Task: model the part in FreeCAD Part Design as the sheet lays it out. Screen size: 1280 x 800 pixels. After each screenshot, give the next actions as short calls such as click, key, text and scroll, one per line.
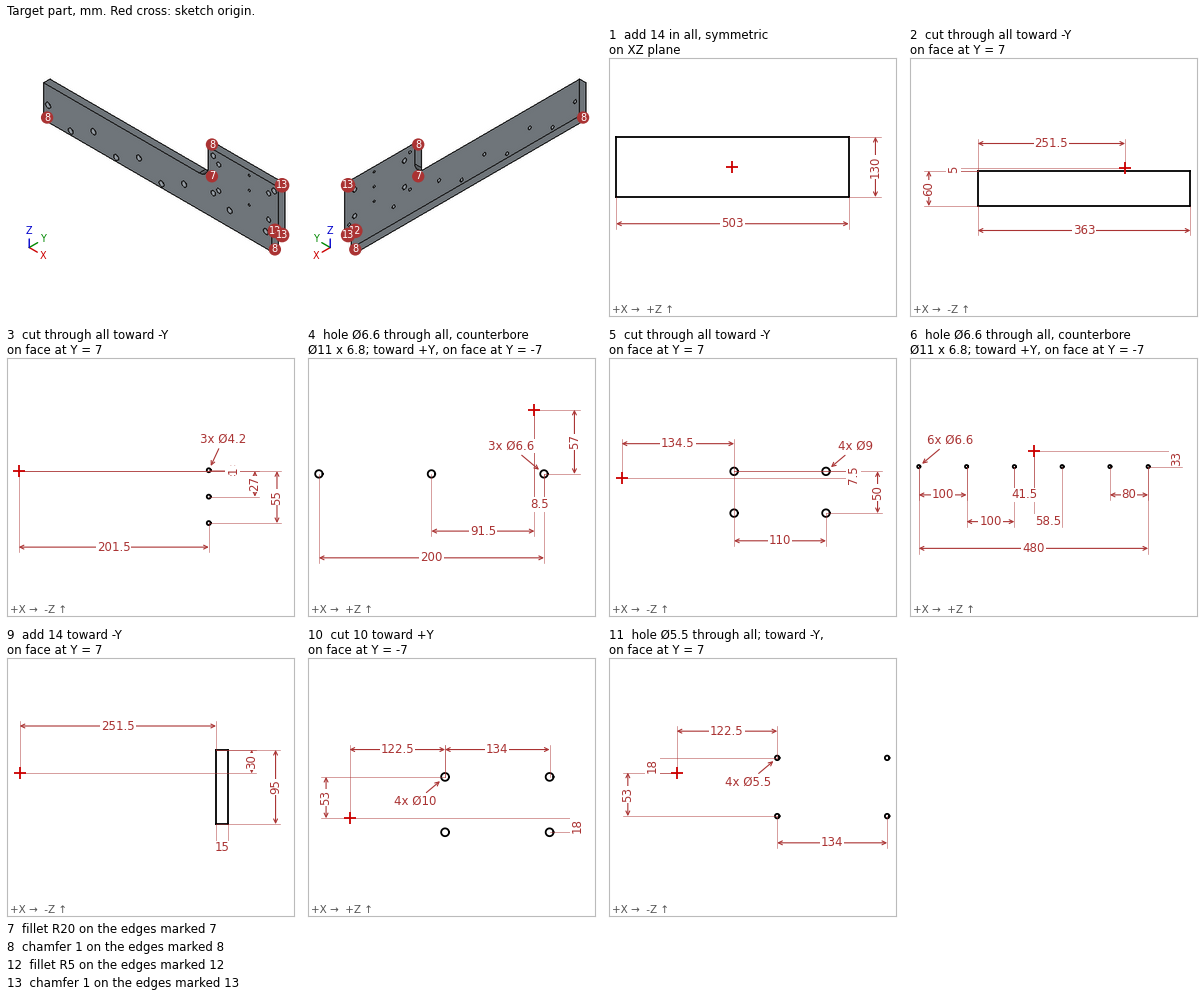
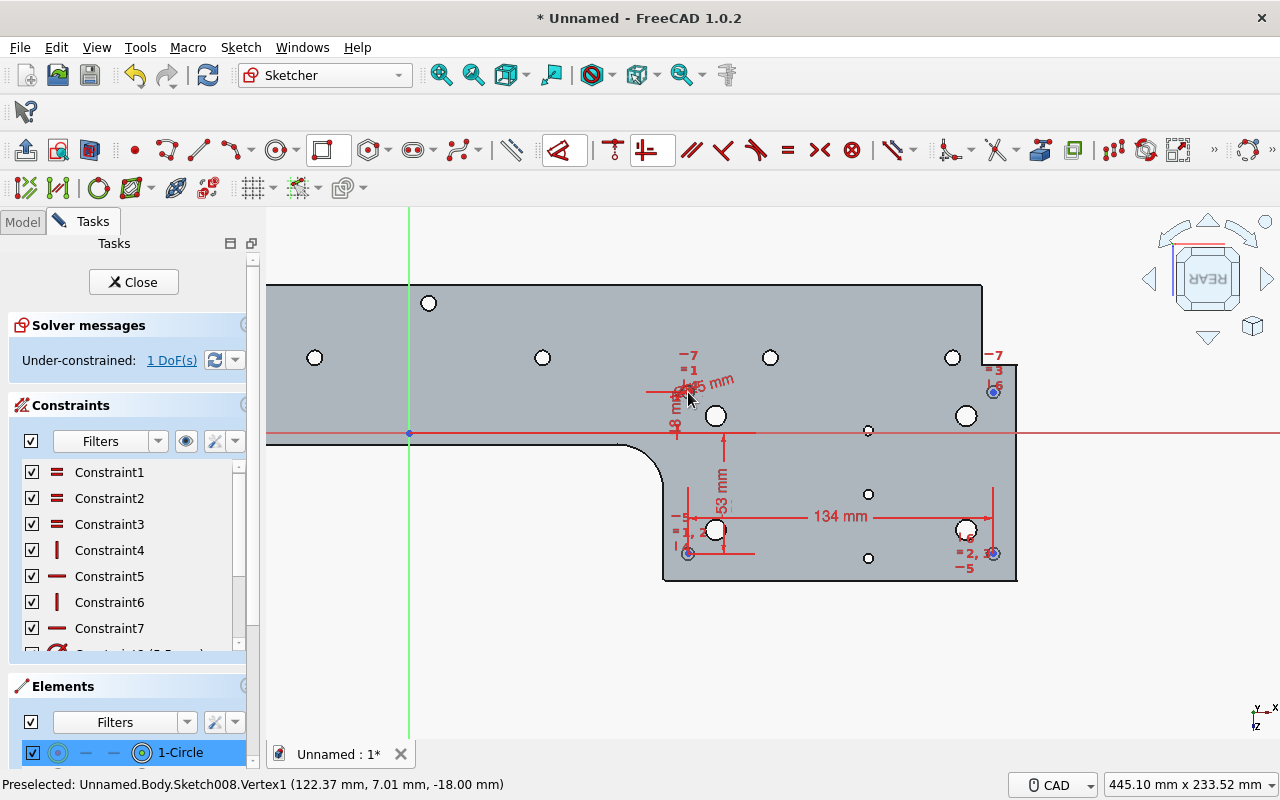
key(l)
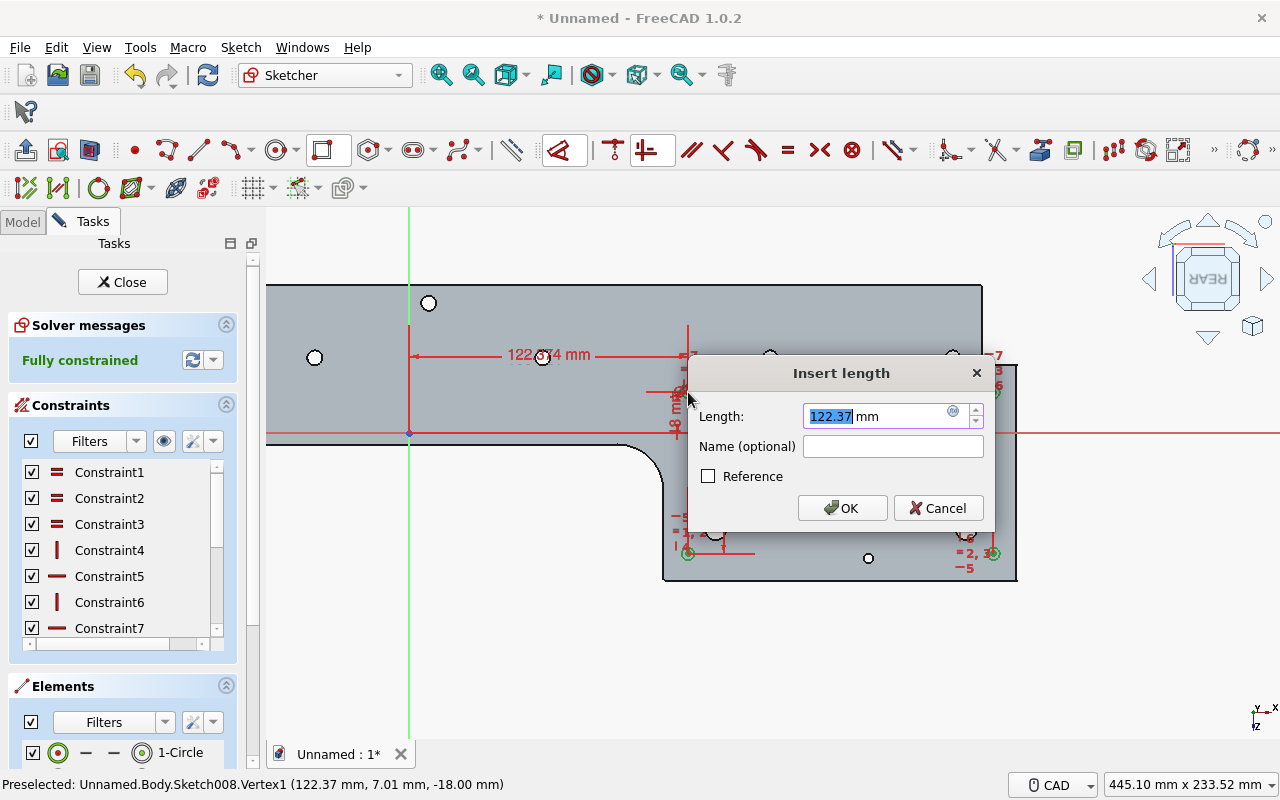
text(122.5)
key(Return)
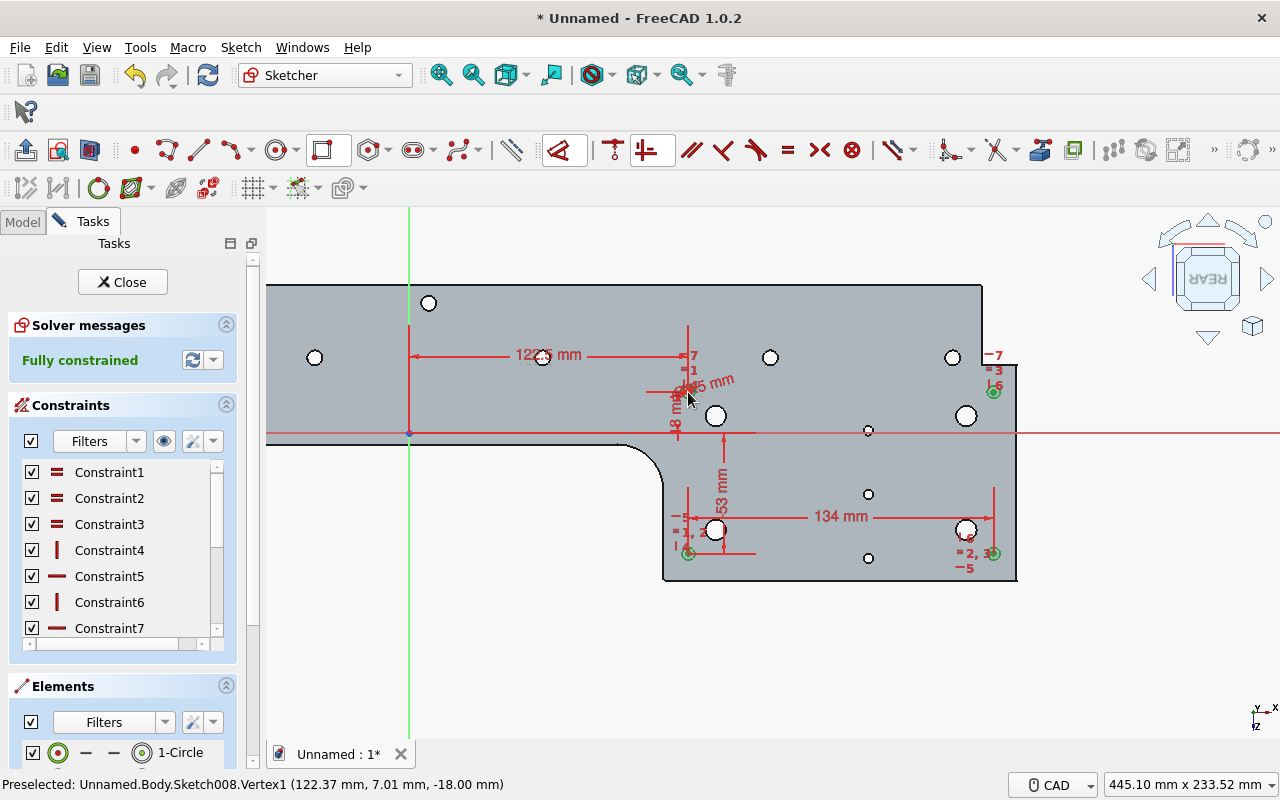
click(123, 282)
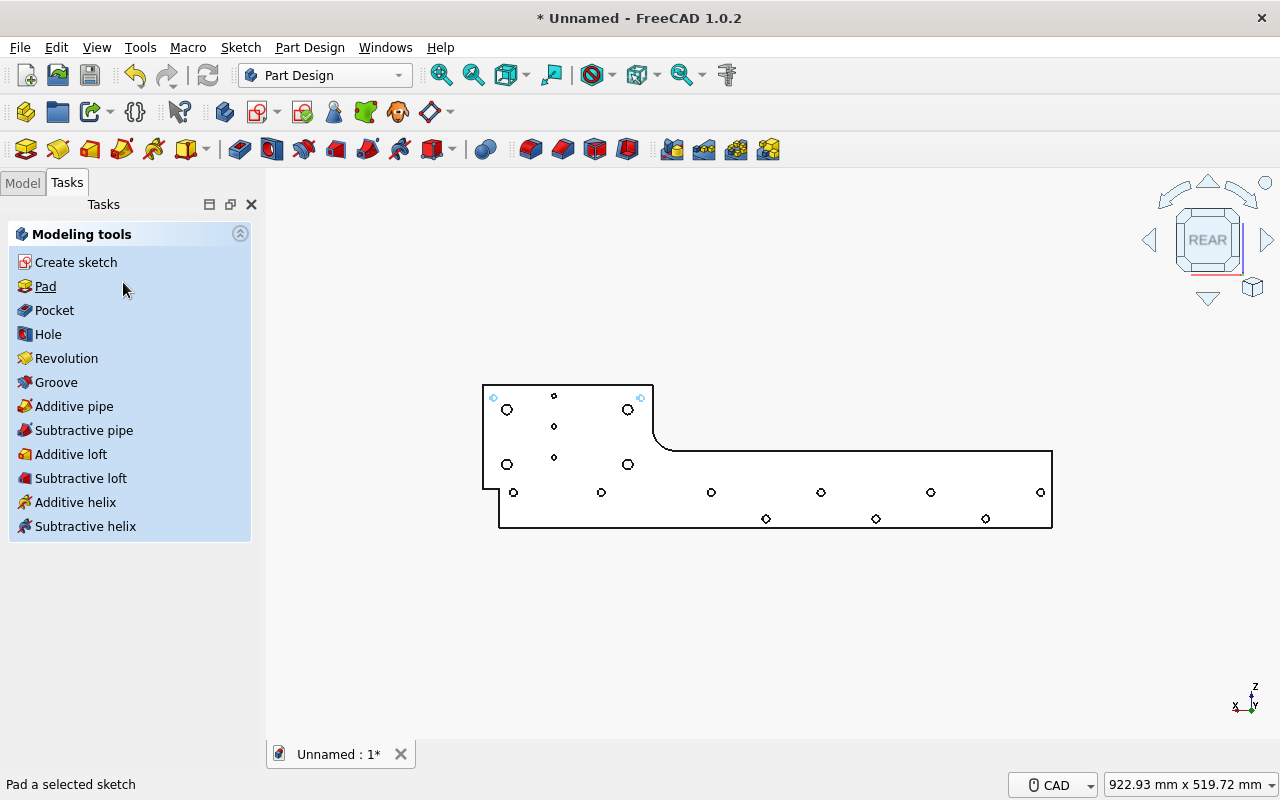
click(272, 150)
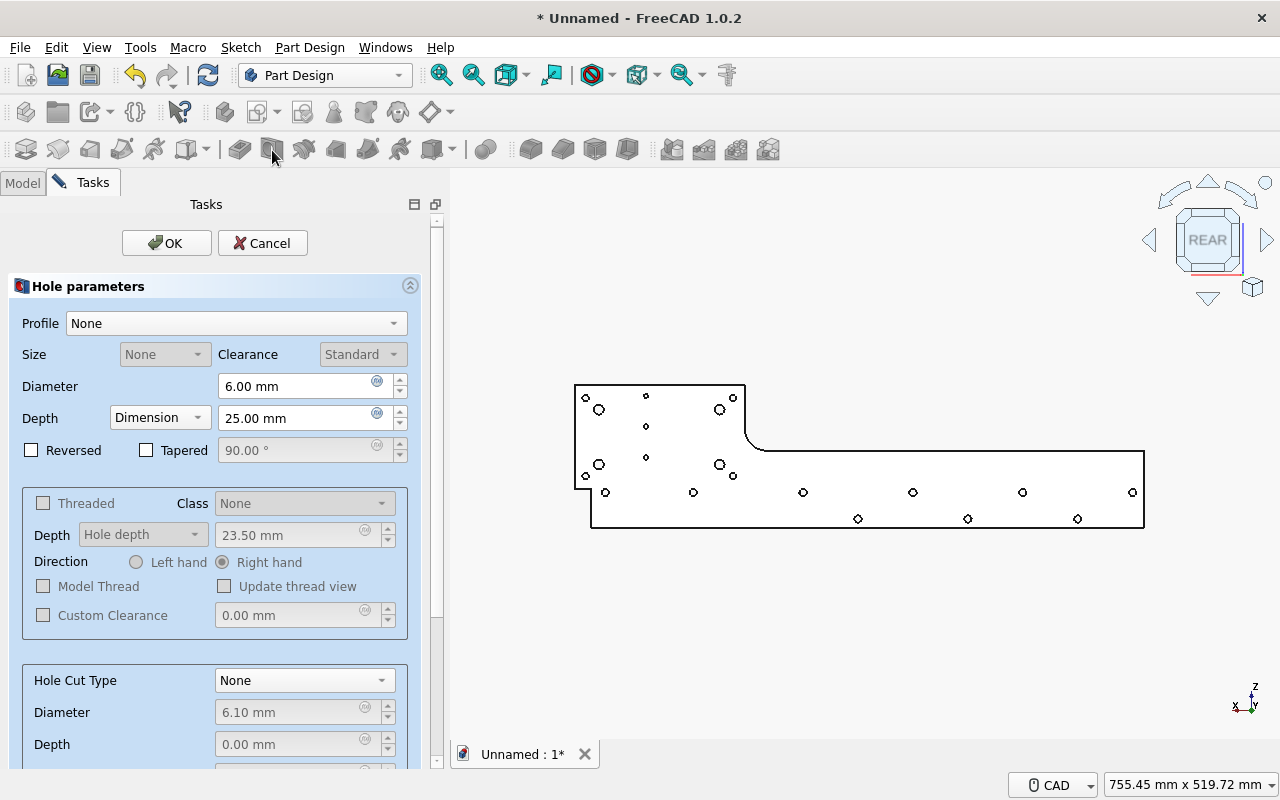
triple_click(305, 386)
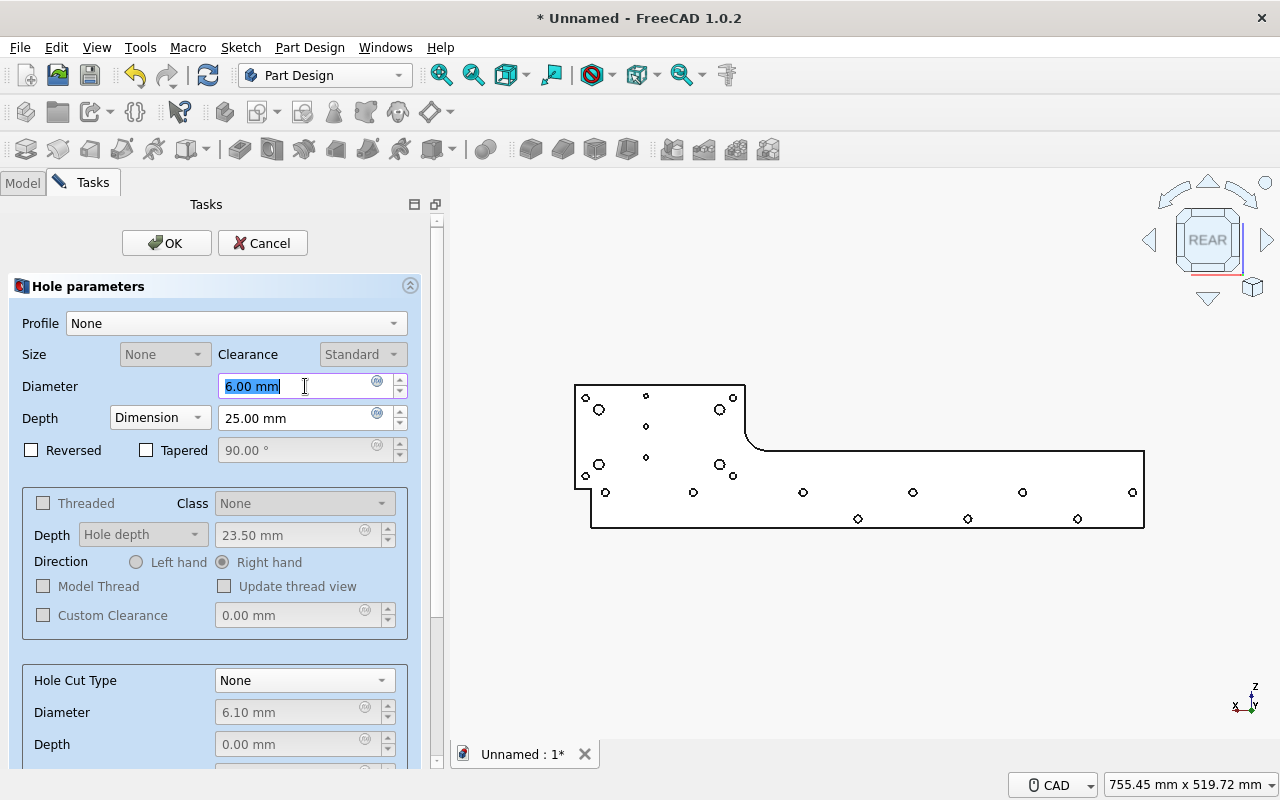
text(5.5)
key(Tab)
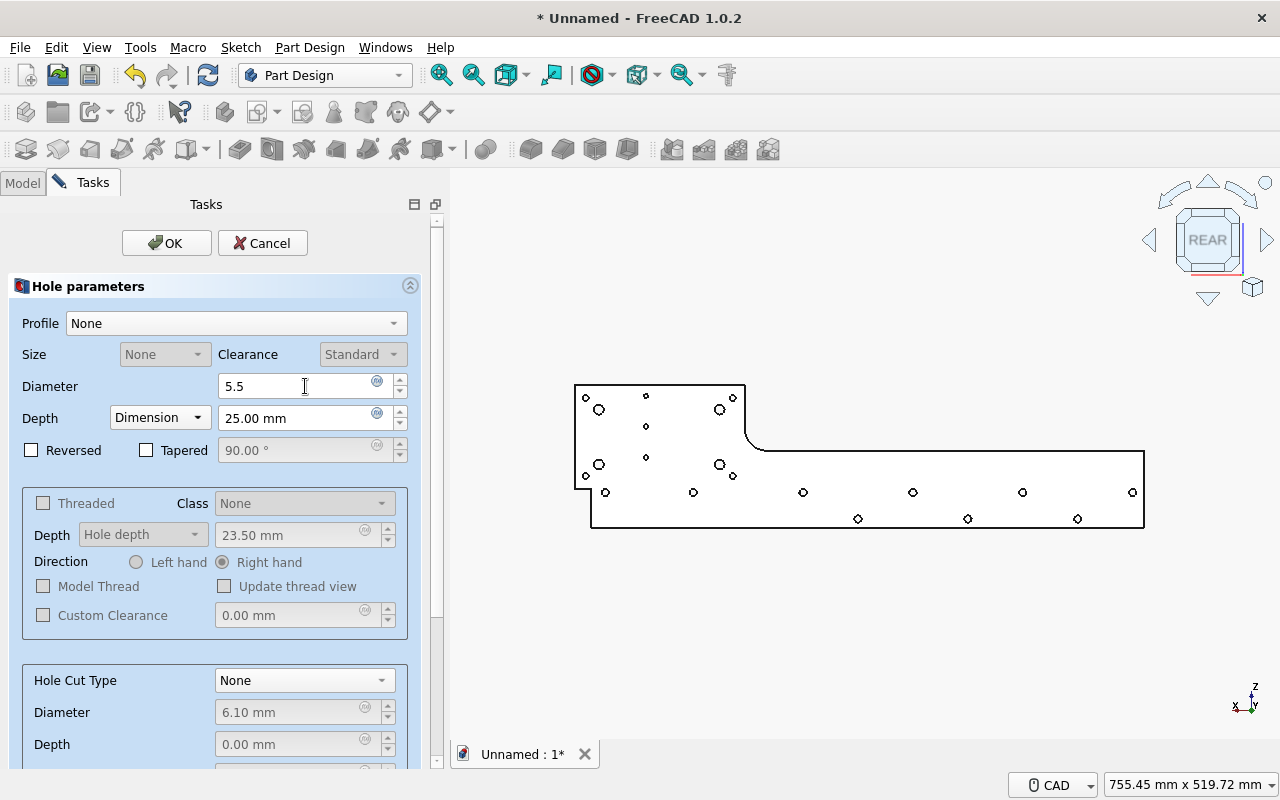
click(161, 418)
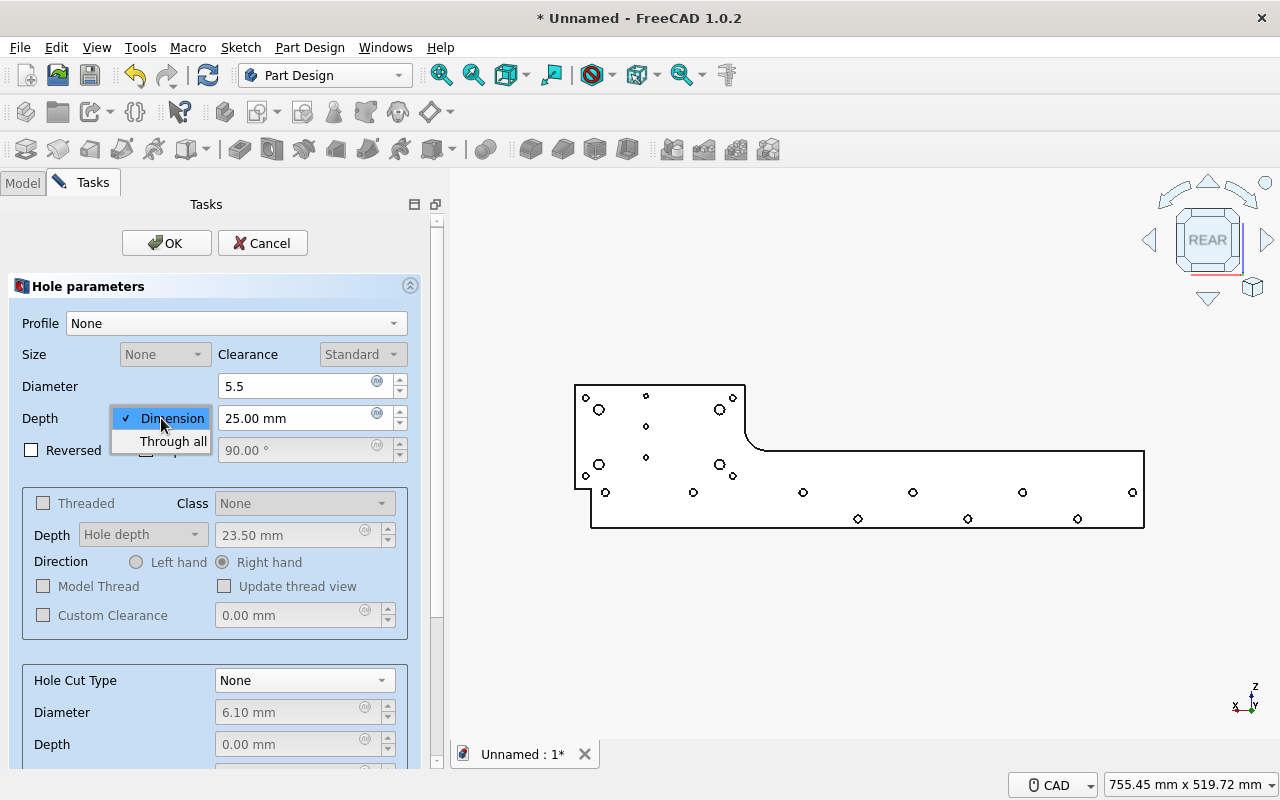
click(160, 442)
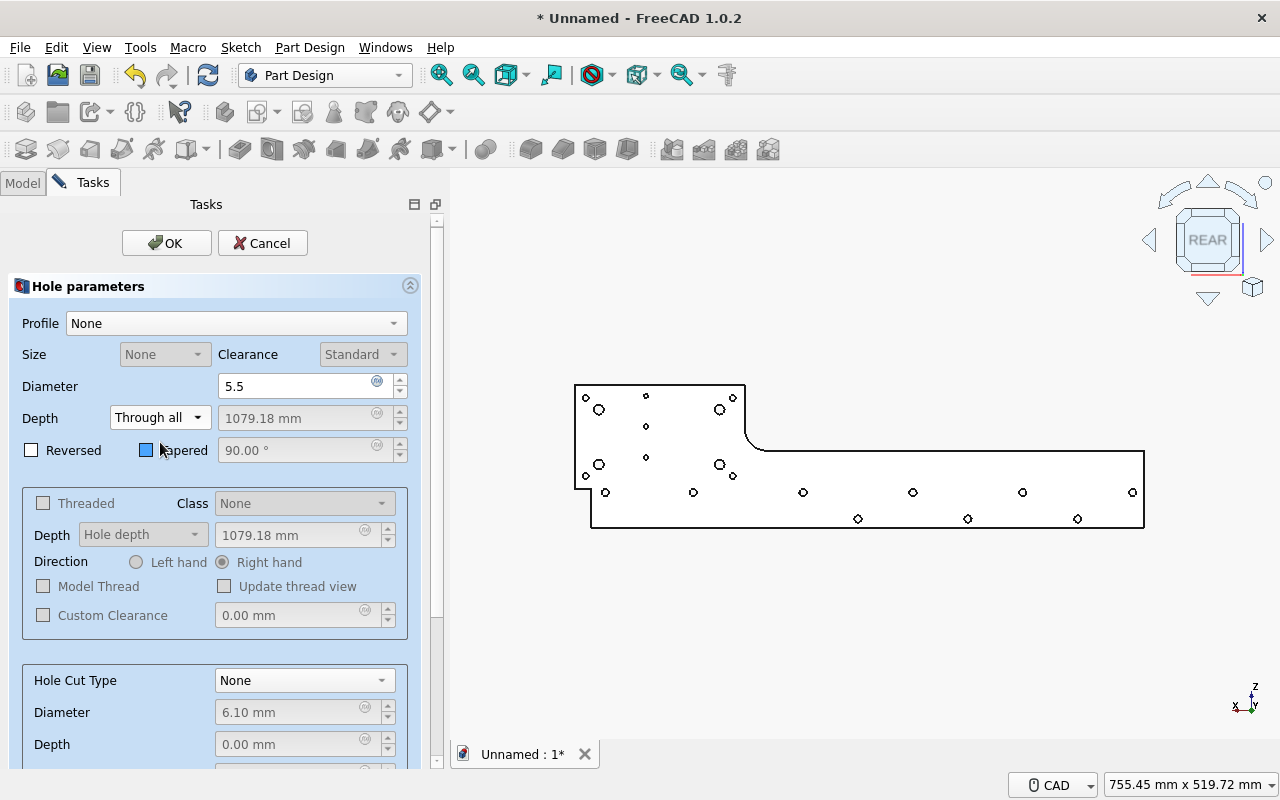
click(167, 243)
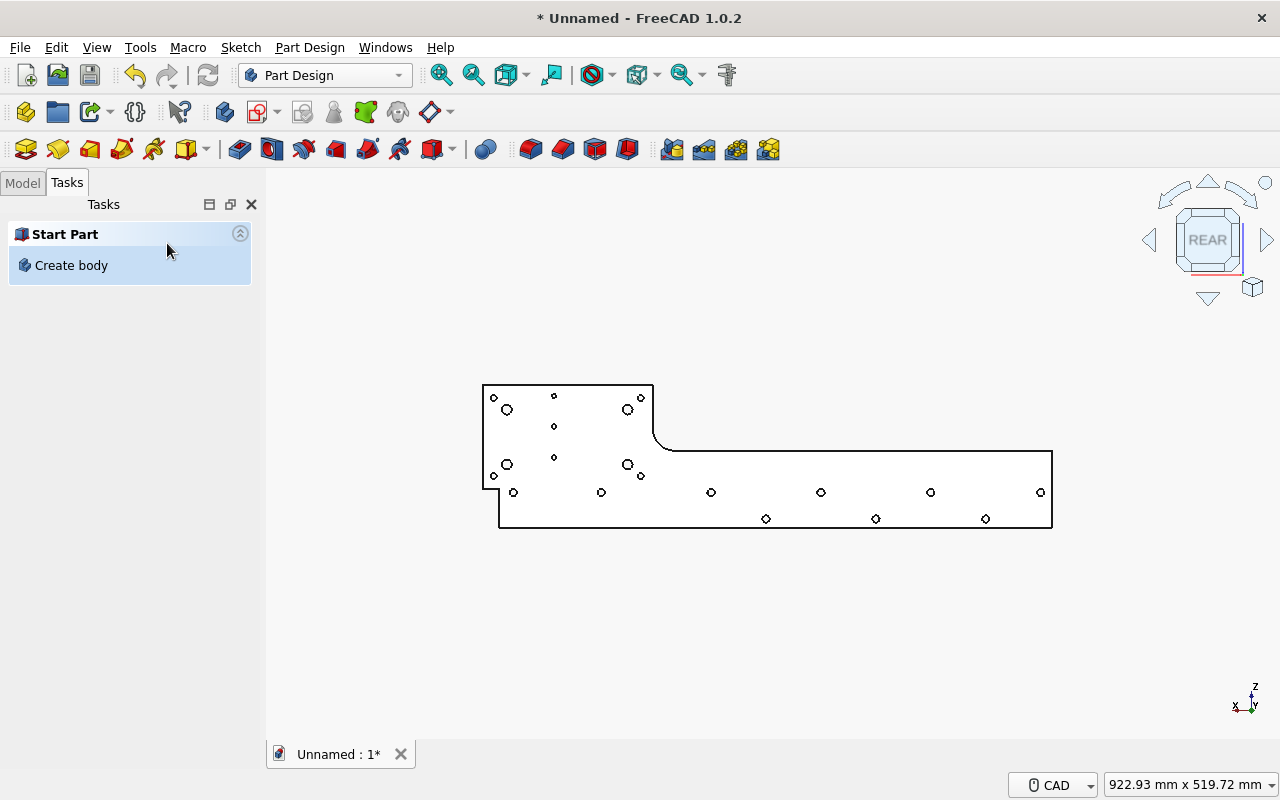
scroll(499, 488, up, 5)